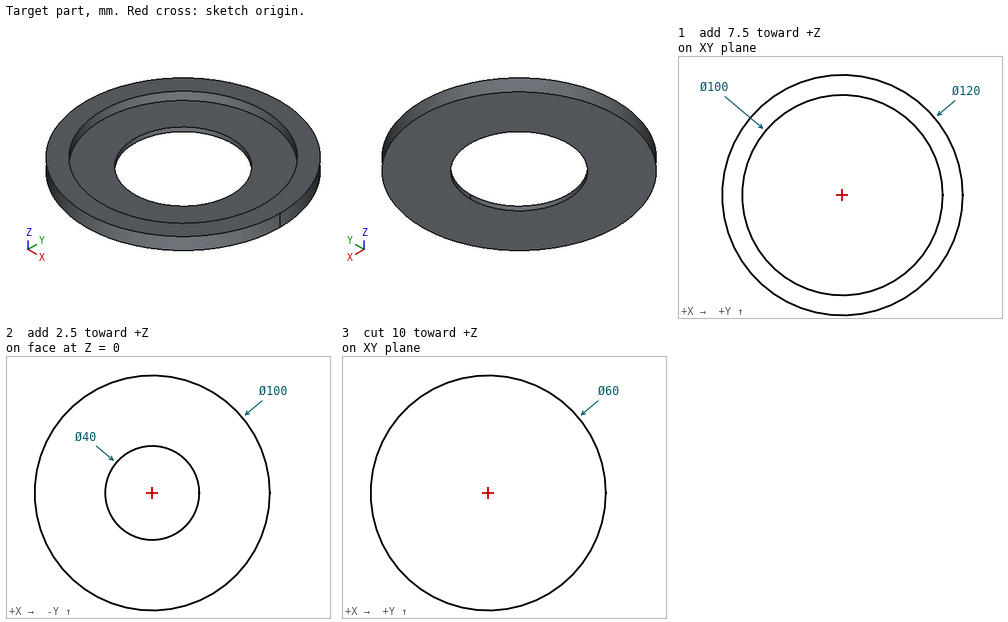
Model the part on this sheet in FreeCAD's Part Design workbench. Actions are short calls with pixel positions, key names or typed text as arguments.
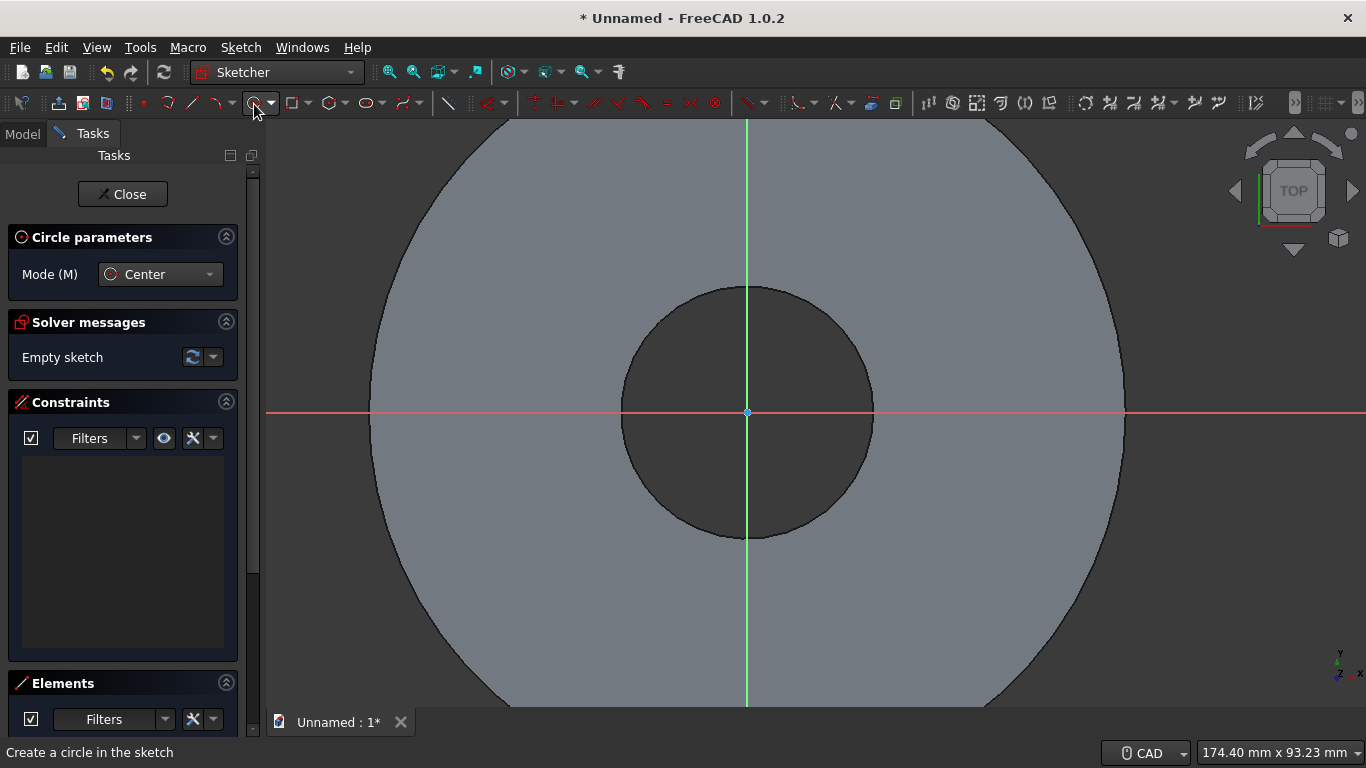
click(747, 413)
click(881, 279)
key(Escape)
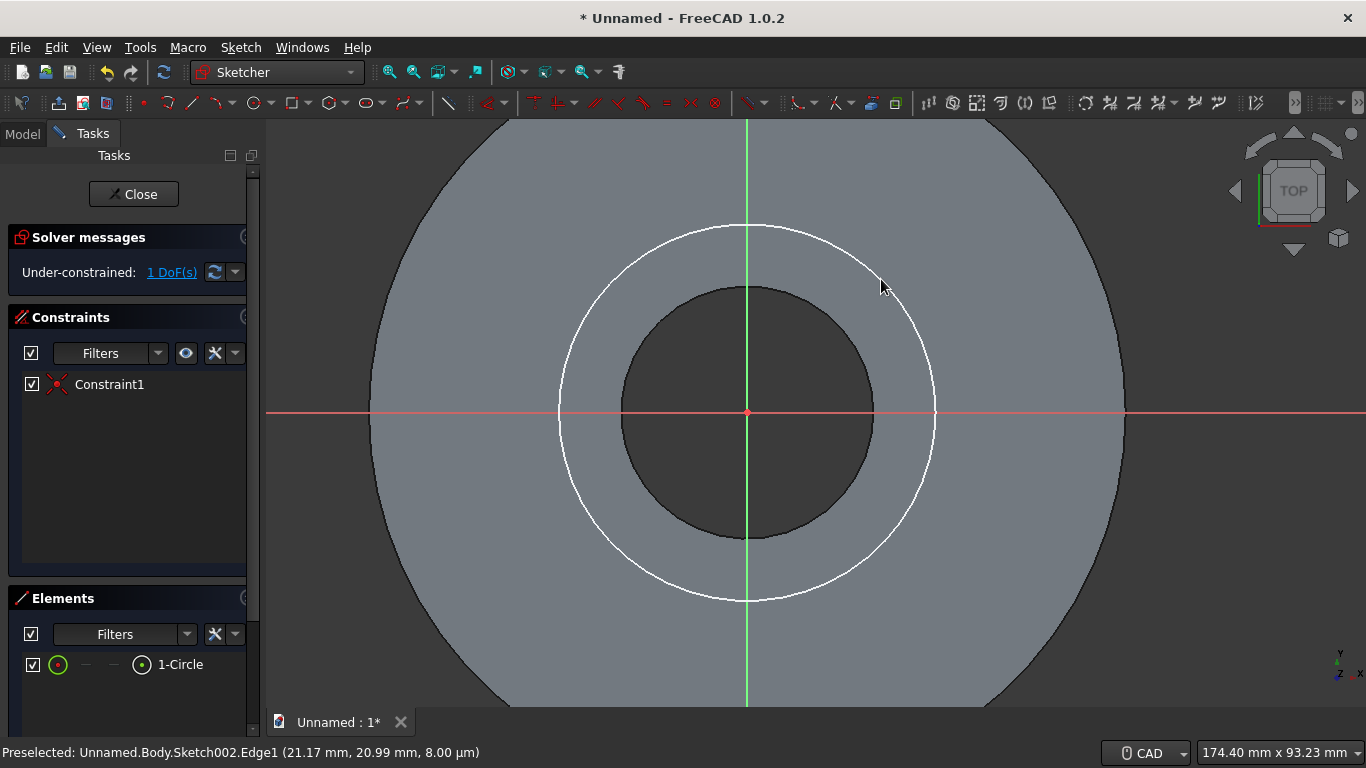
click(488, 104)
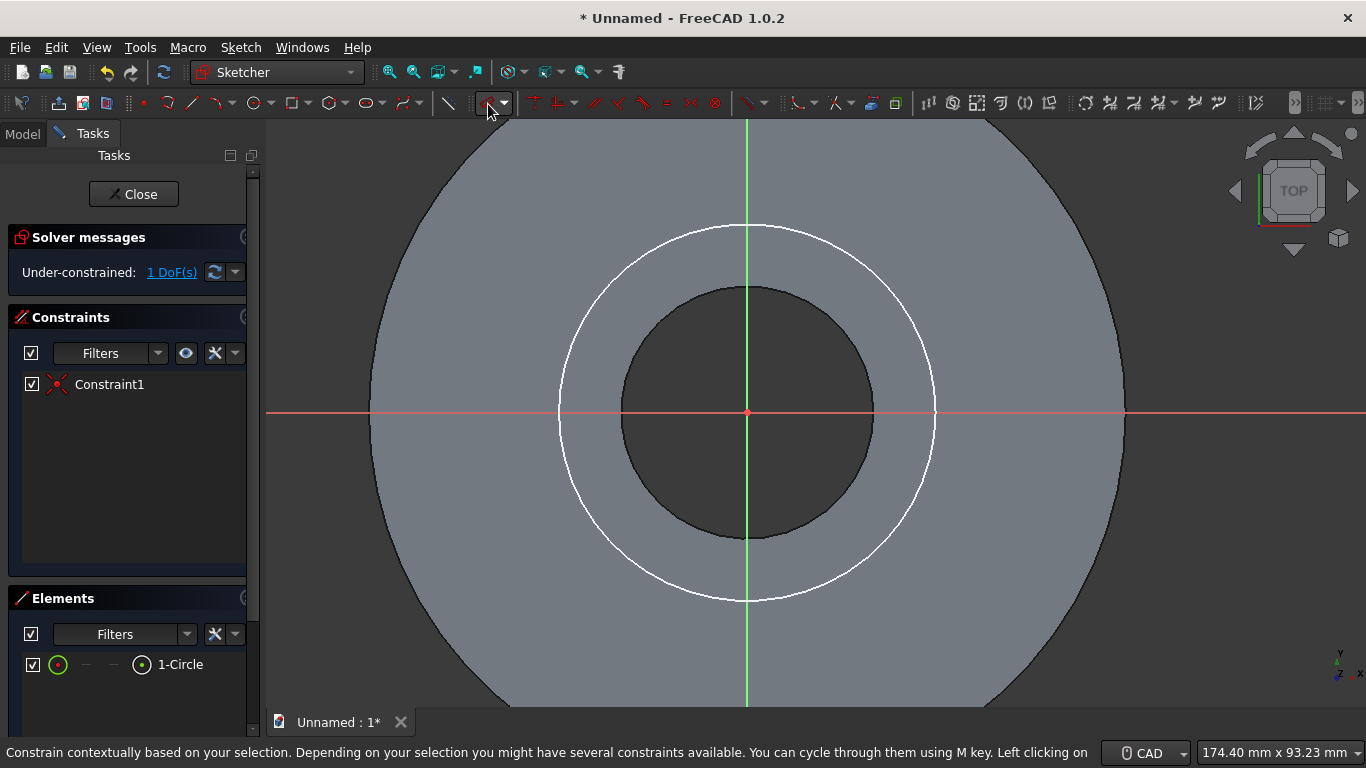
click(880, 279)
click(903, 256)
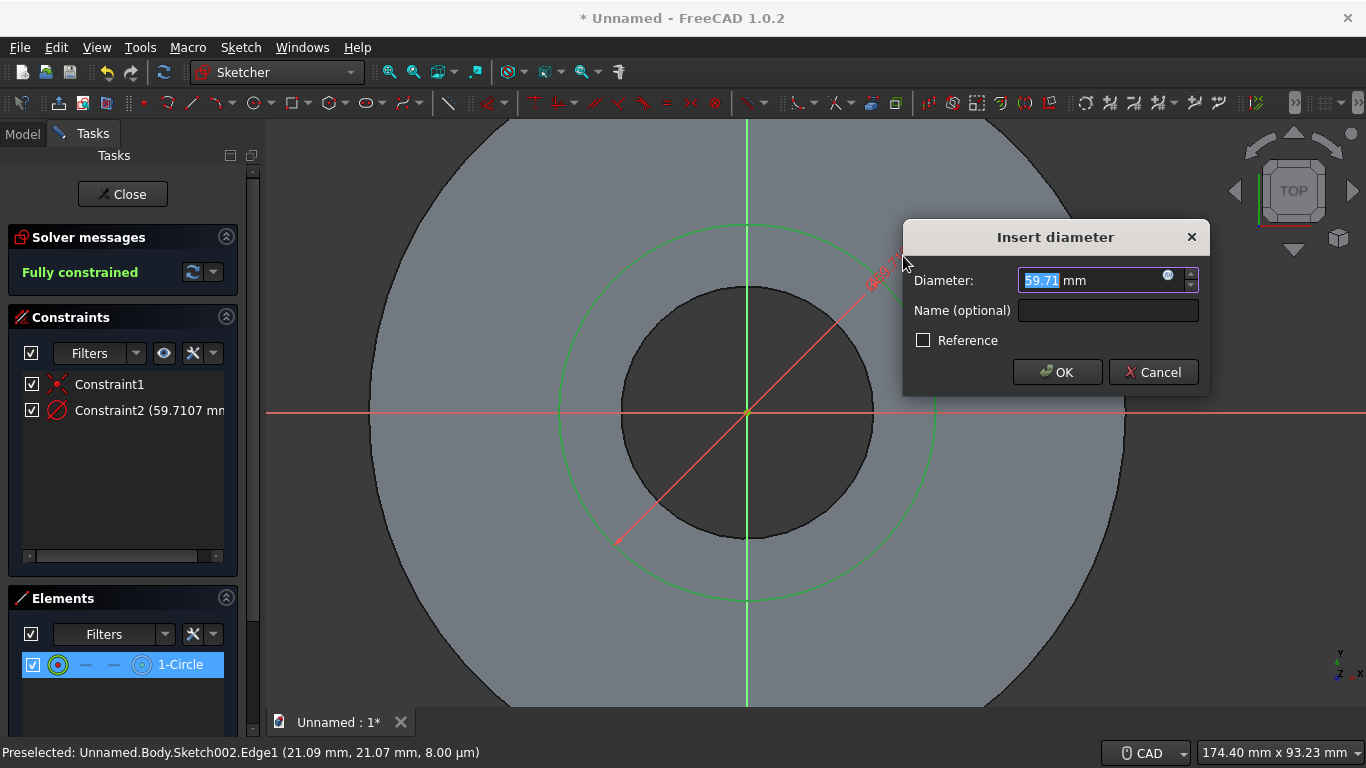
text(60)
key(Return)
key(Escape)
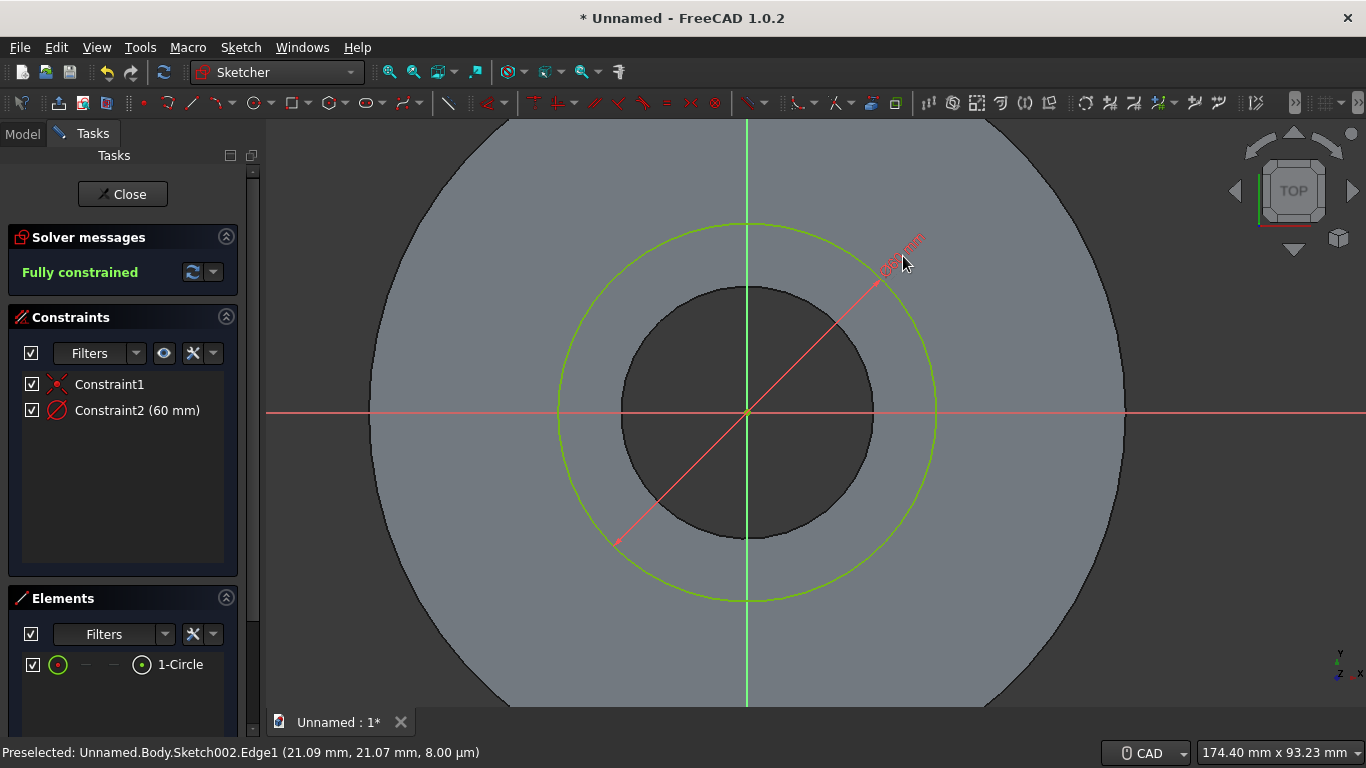
click(123, 194)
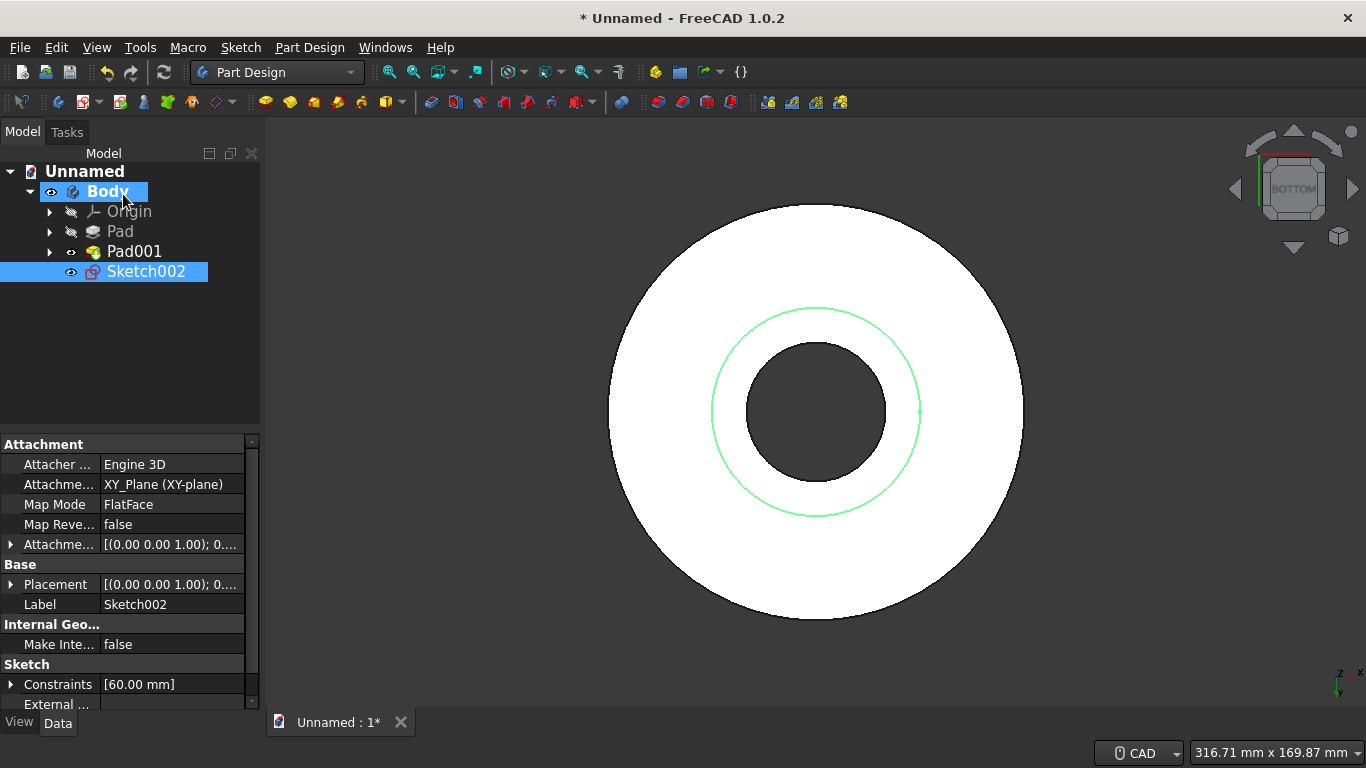
click(432, 102)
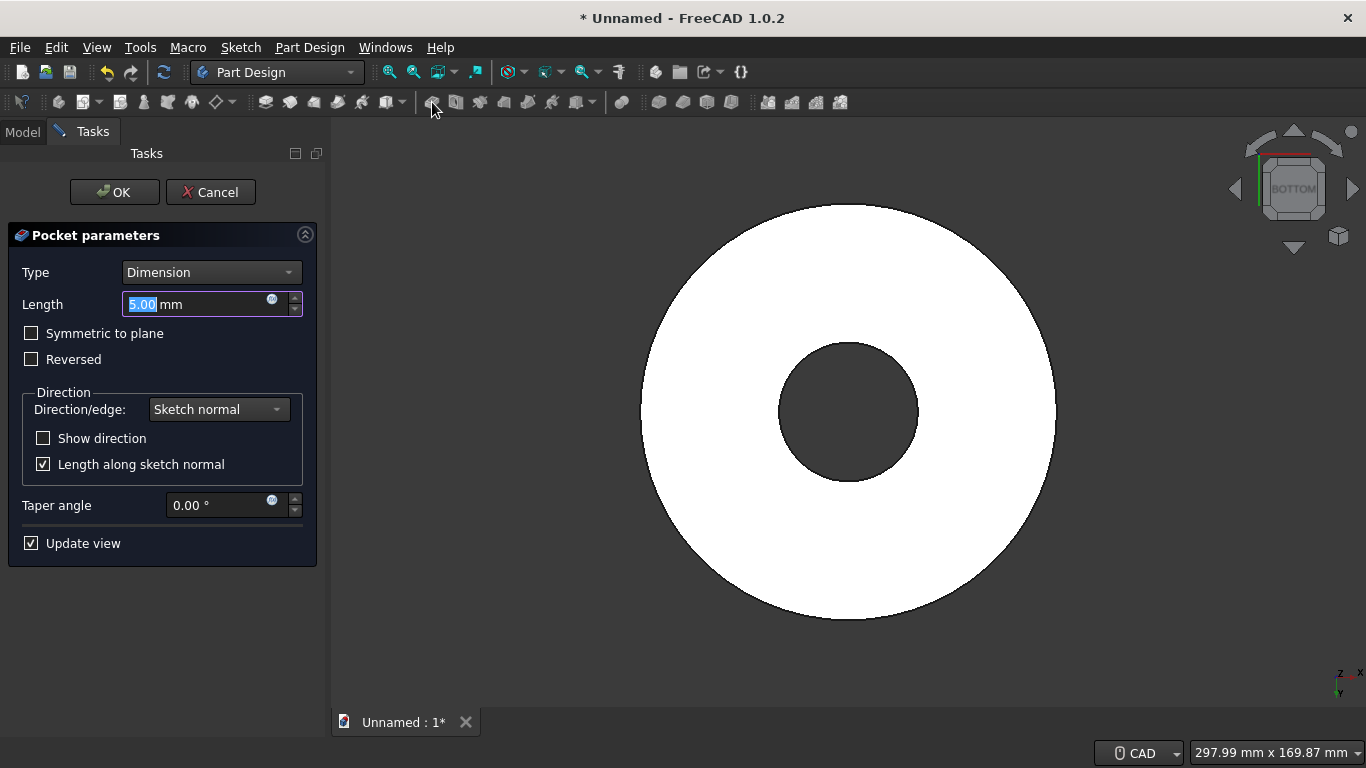
text(10)
key(Tab)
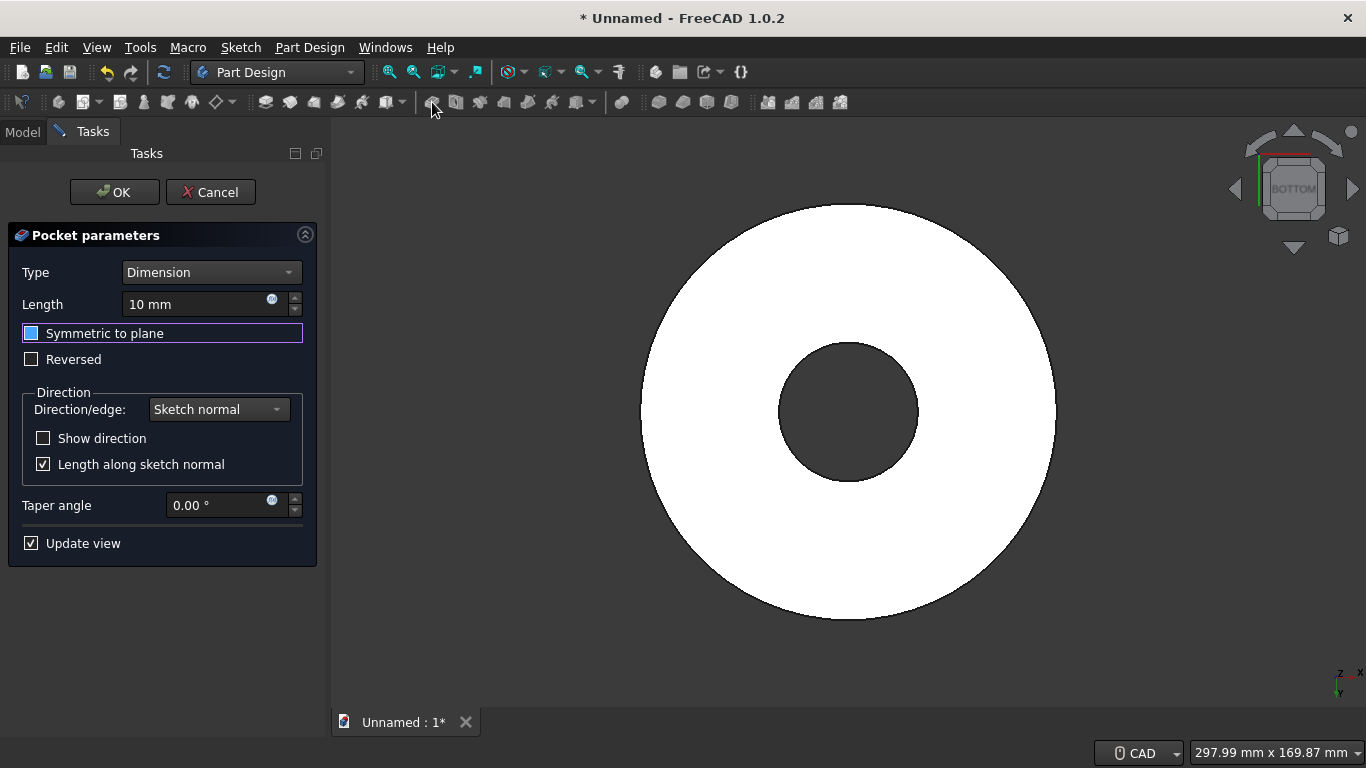
click(30, 359)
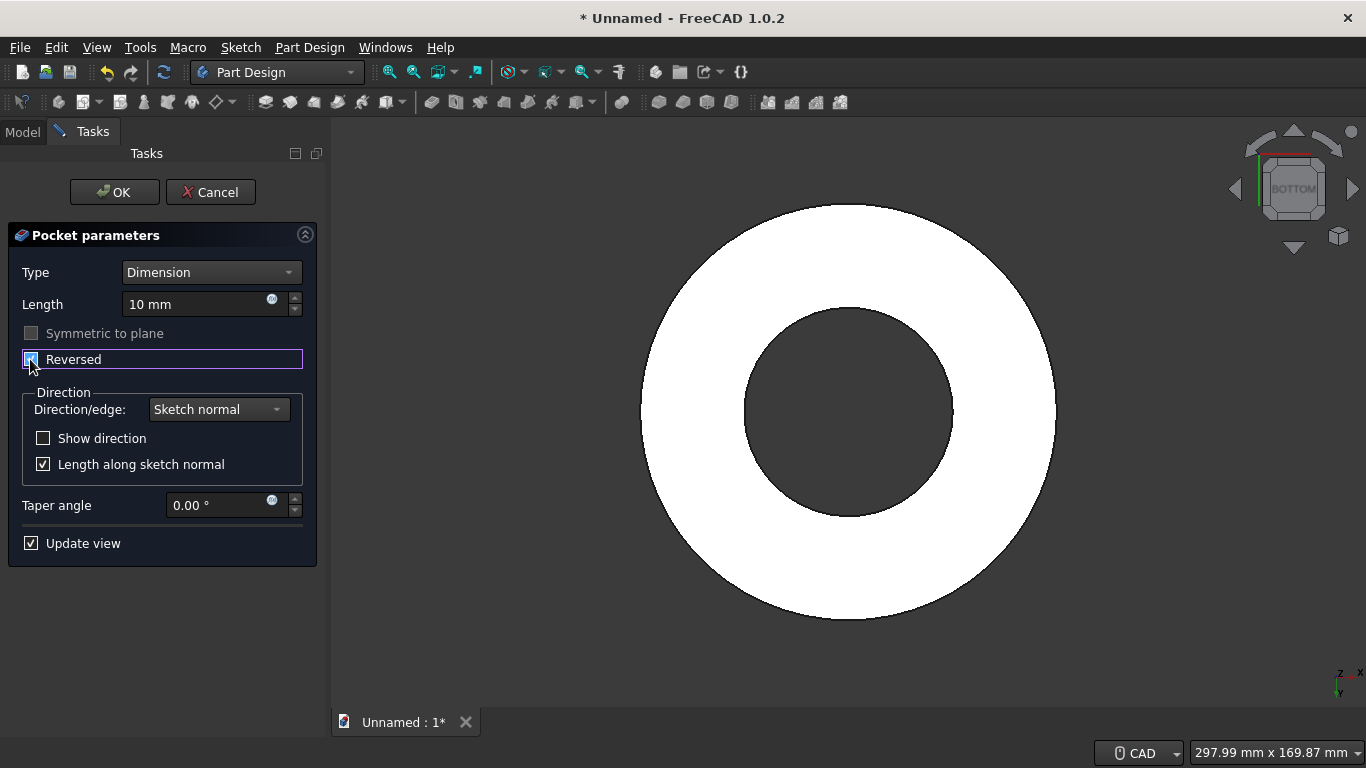
click(115, 192)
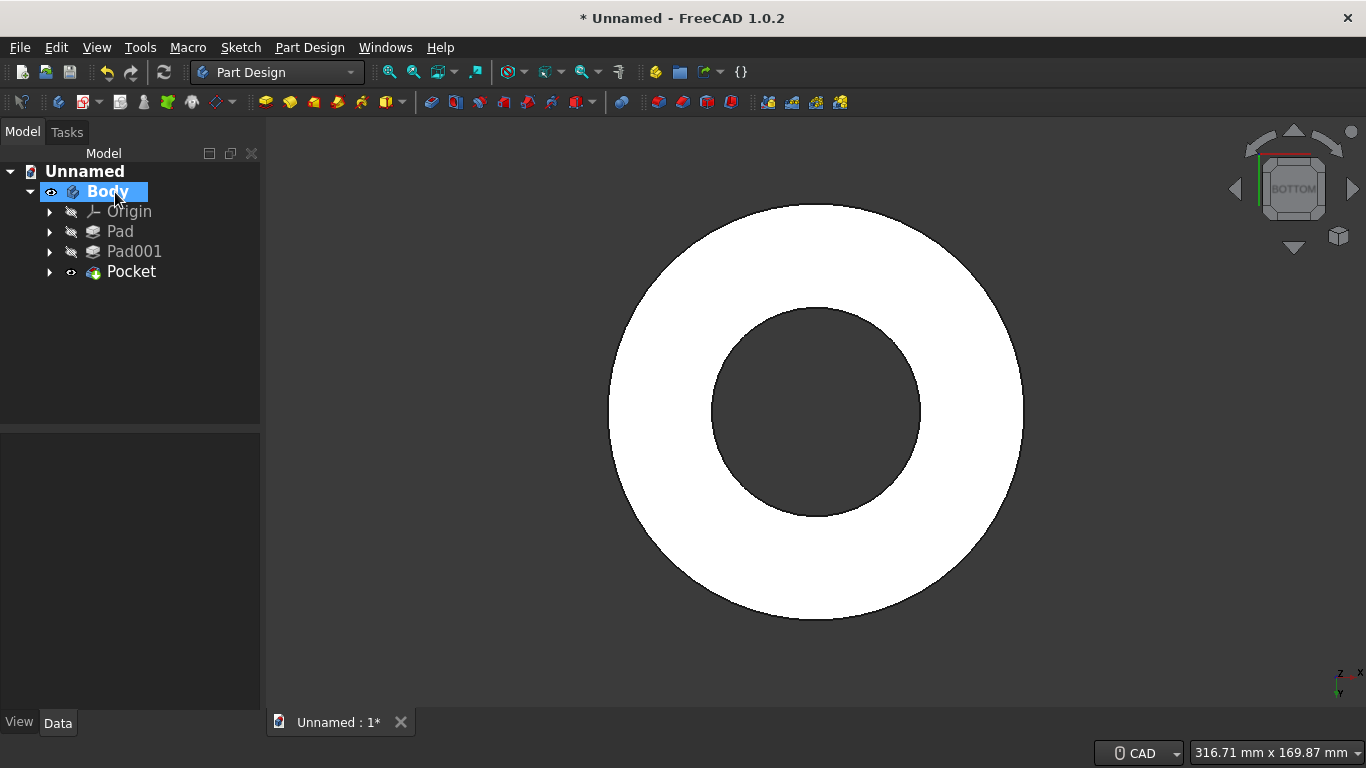
key(0)